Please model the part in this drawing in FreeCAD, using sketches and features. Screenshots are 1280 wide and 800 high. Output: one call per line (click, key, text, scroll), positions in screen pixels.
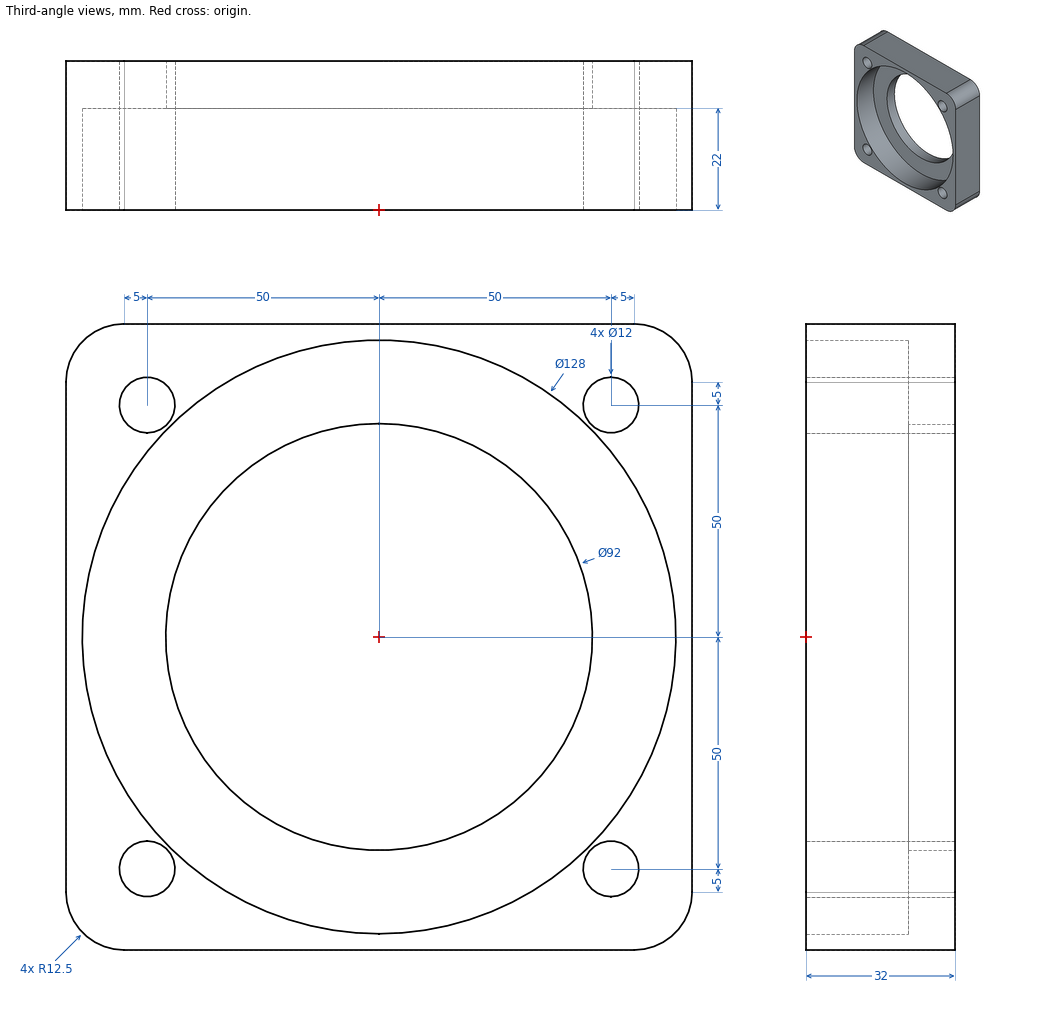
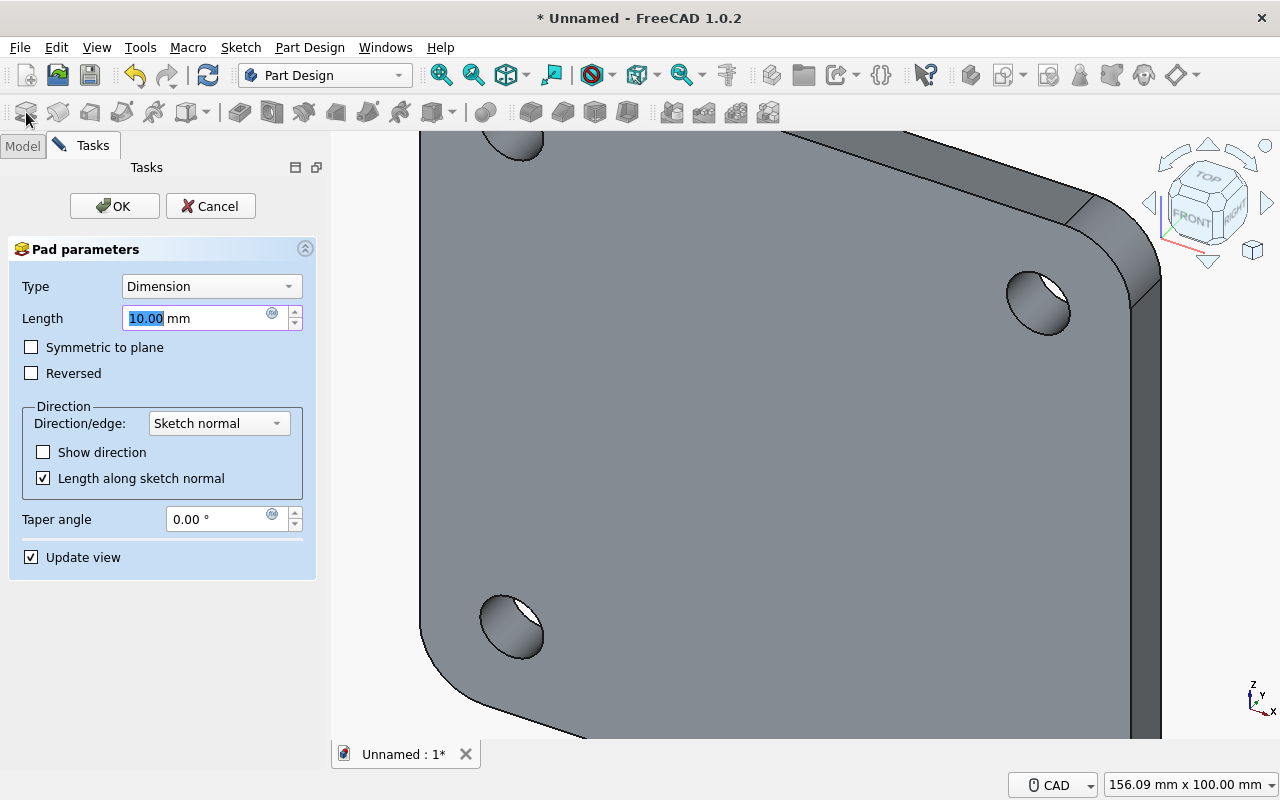
text(32)
key(Tab)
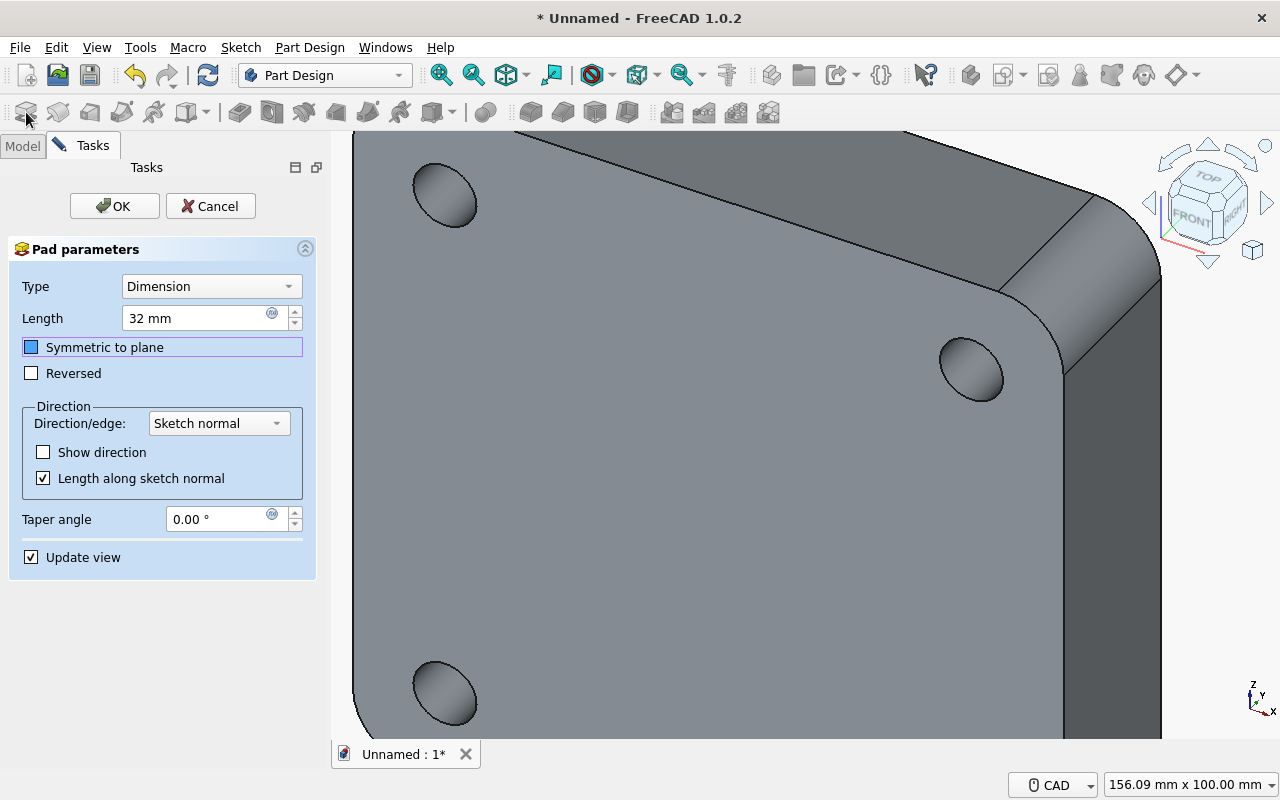
click(30, 373)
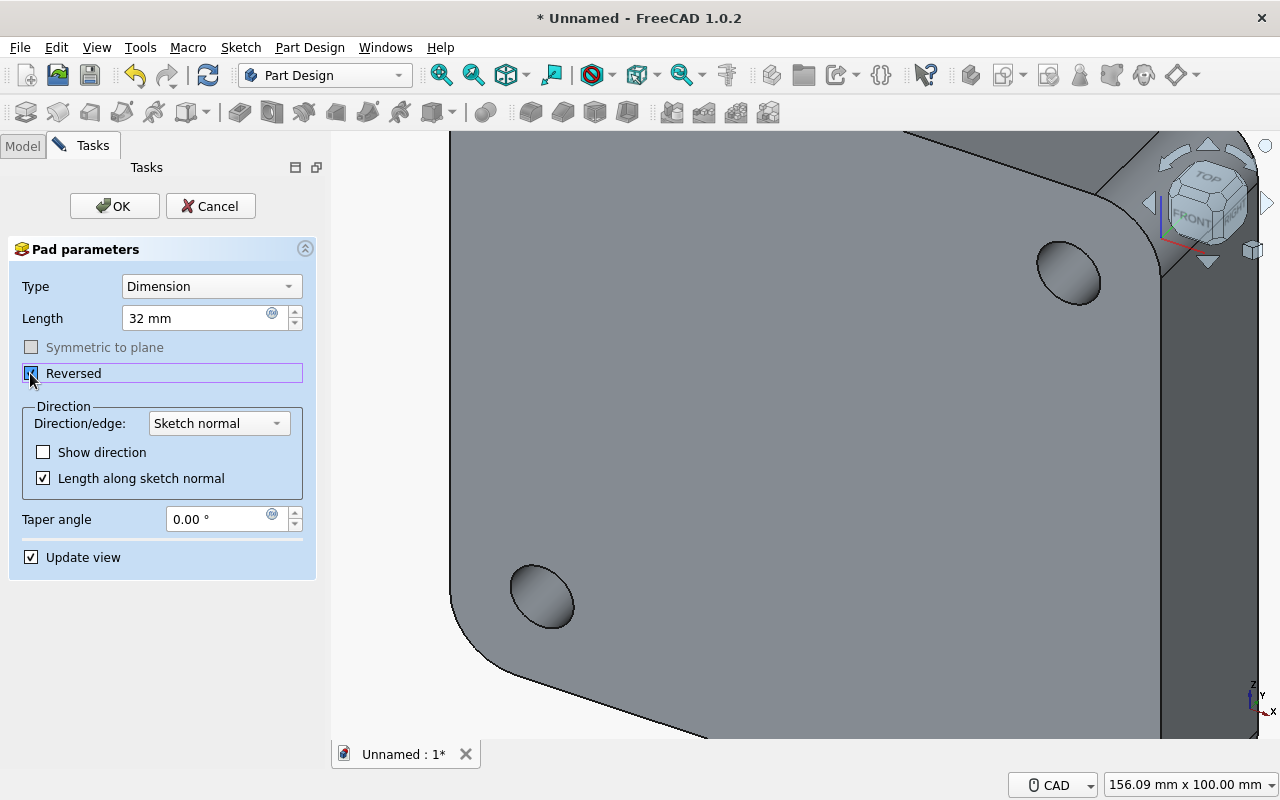
click(115, 206)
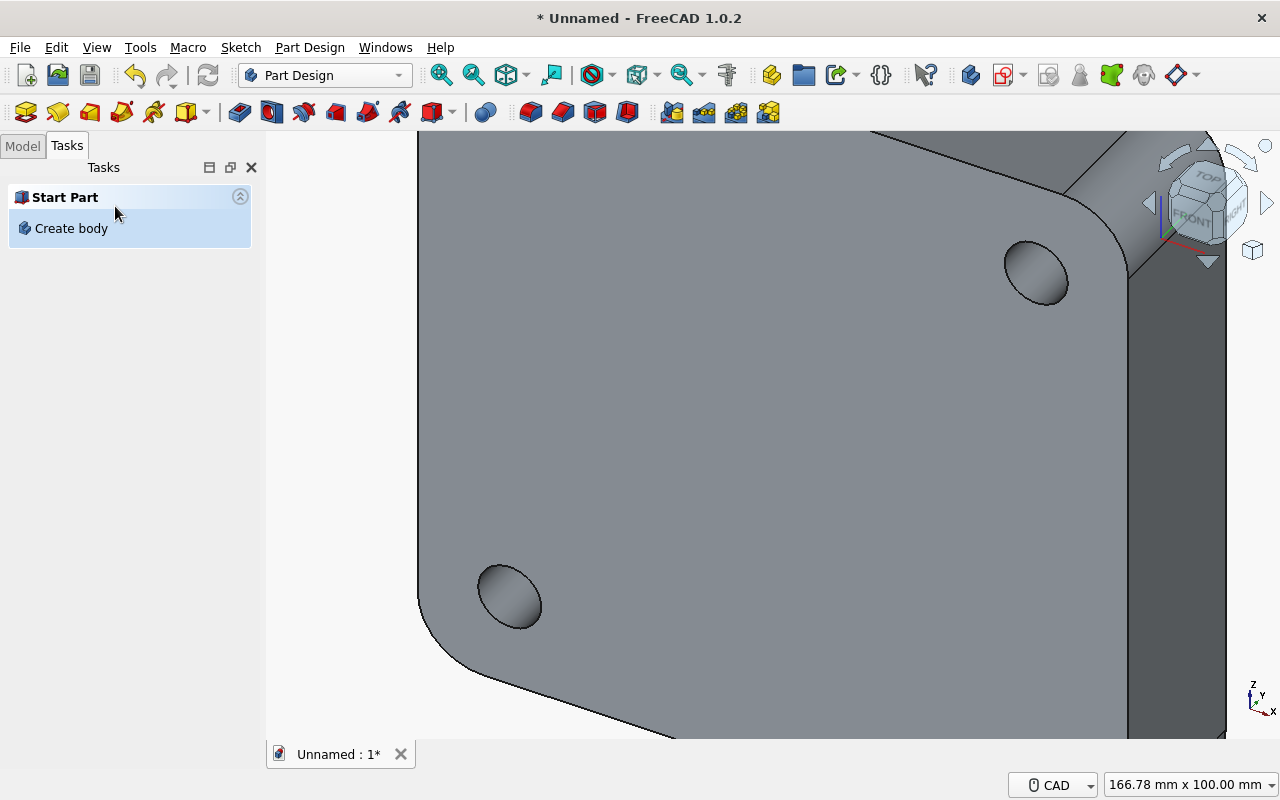
click(442, 76)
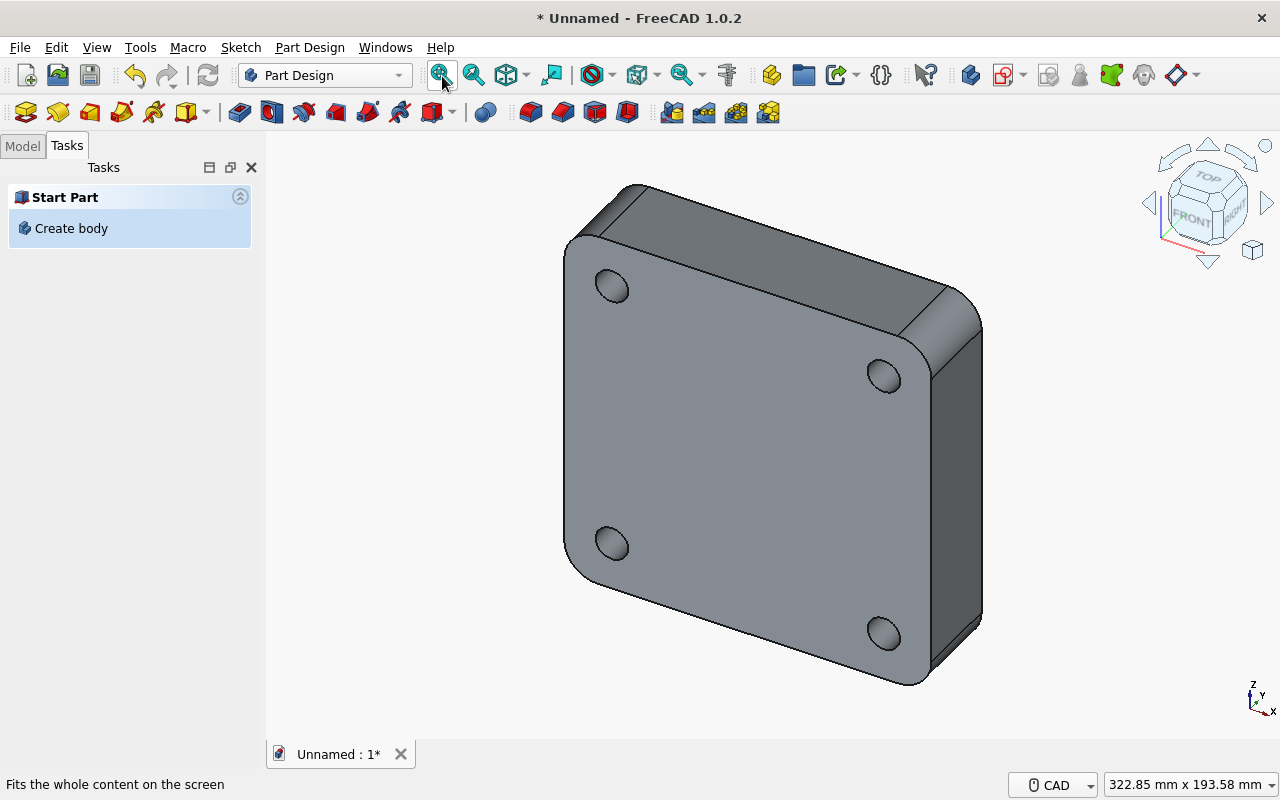
key(4)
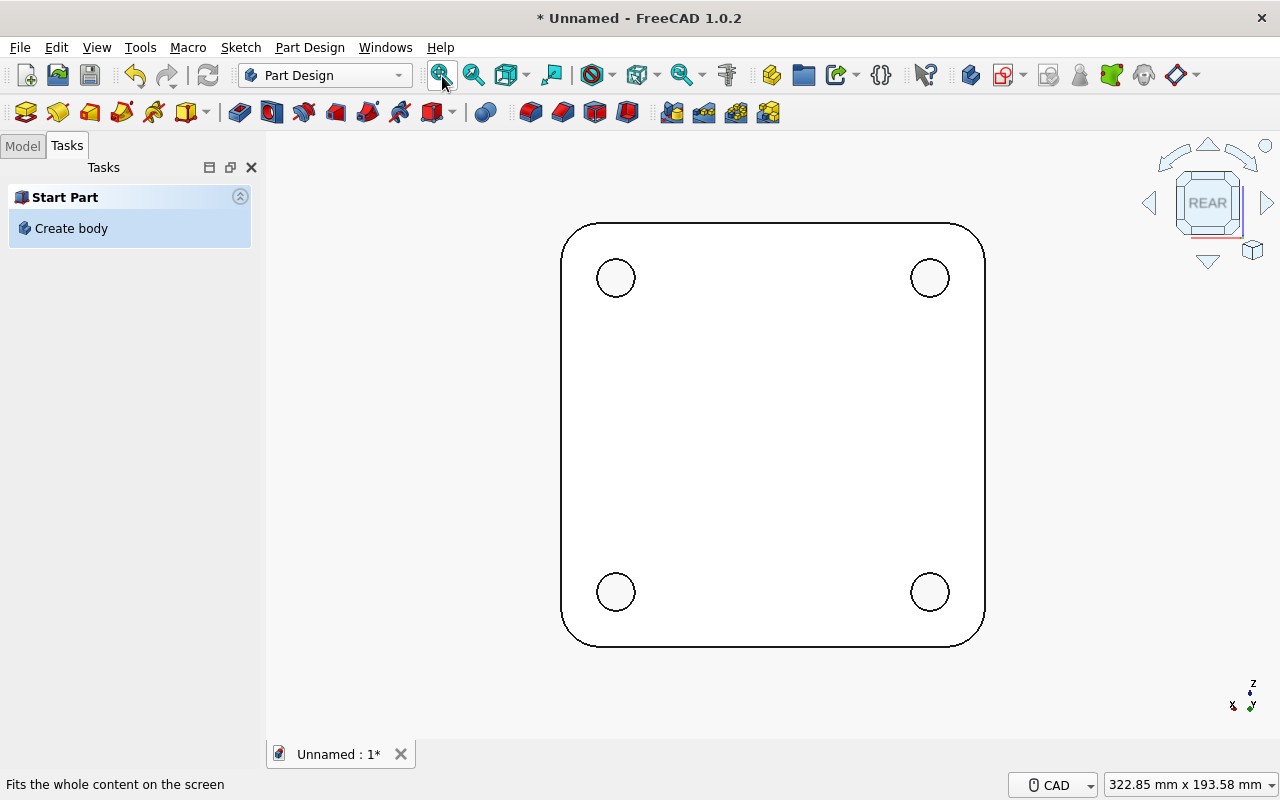
click(773, 434)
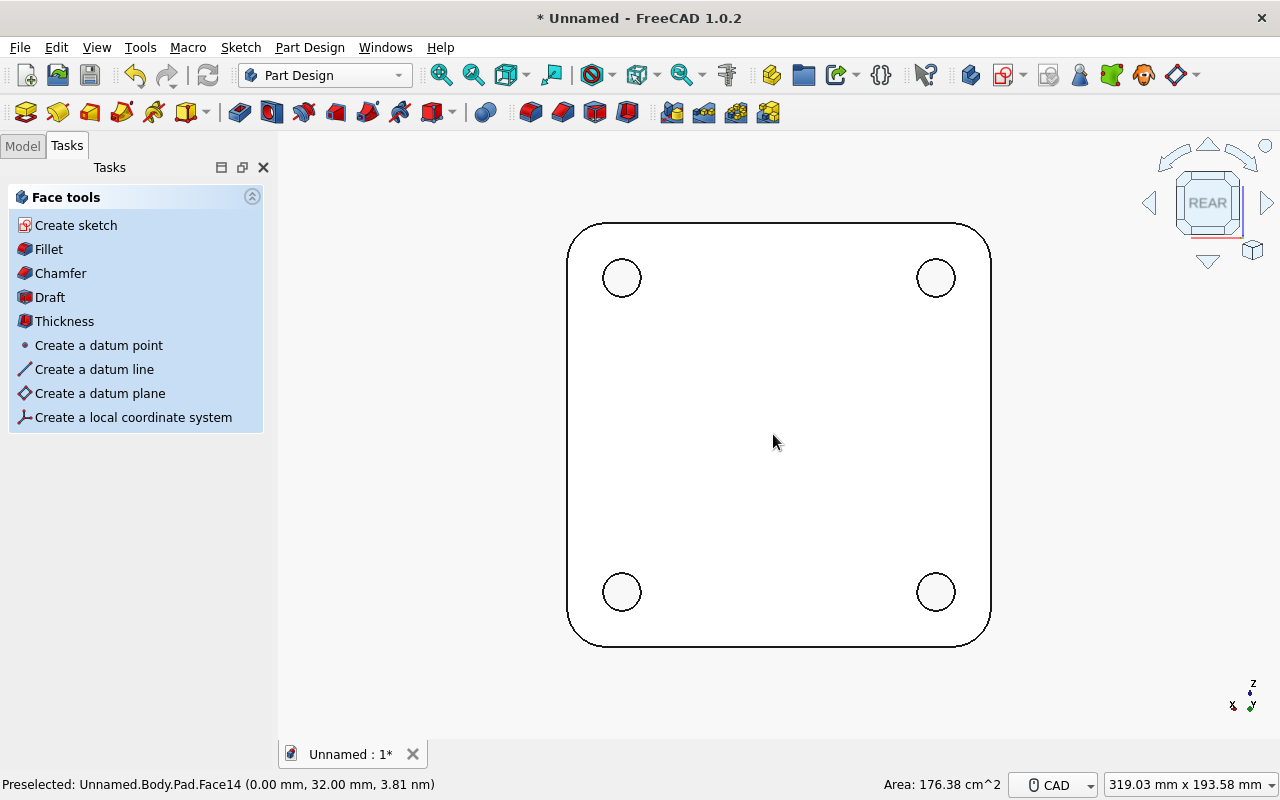
click(1004, 76)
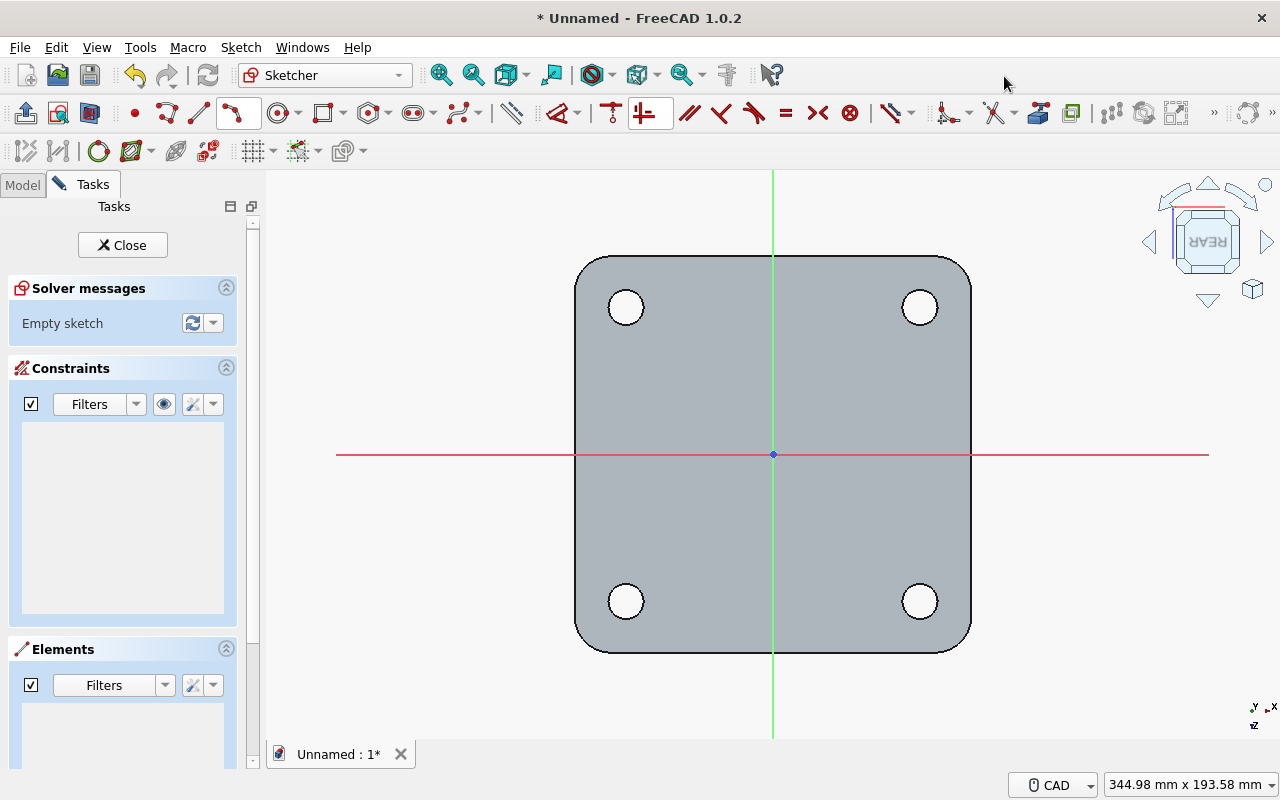
click(278, 114)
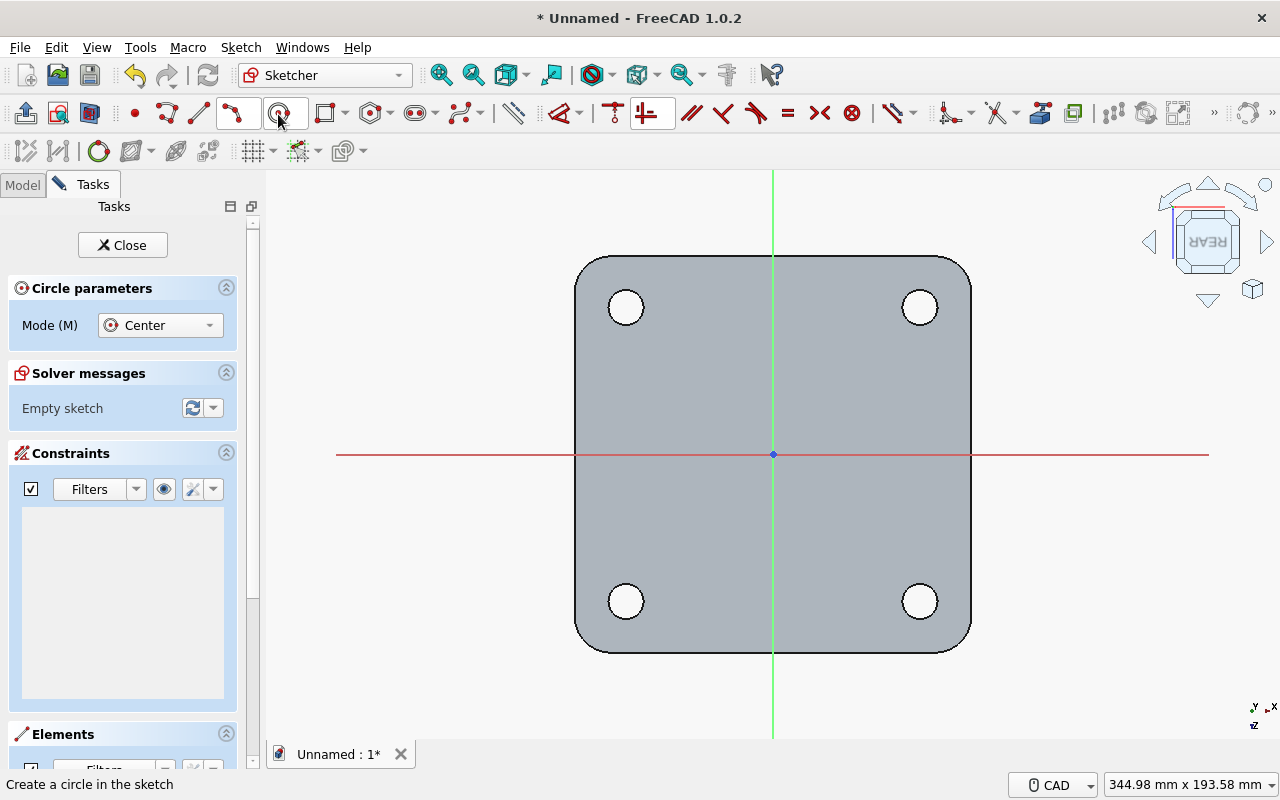
click(773, 455)
click(869, 359)
key(Escape)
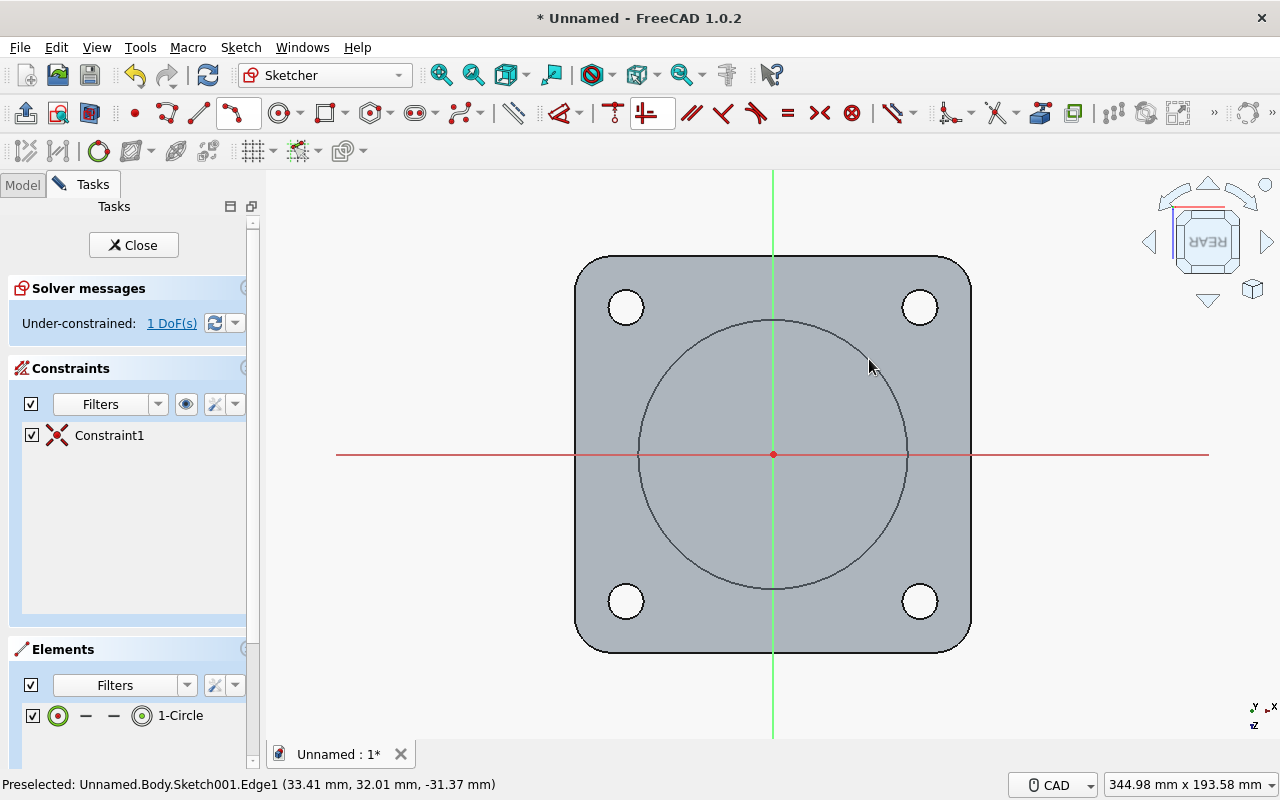
click(560, 114)